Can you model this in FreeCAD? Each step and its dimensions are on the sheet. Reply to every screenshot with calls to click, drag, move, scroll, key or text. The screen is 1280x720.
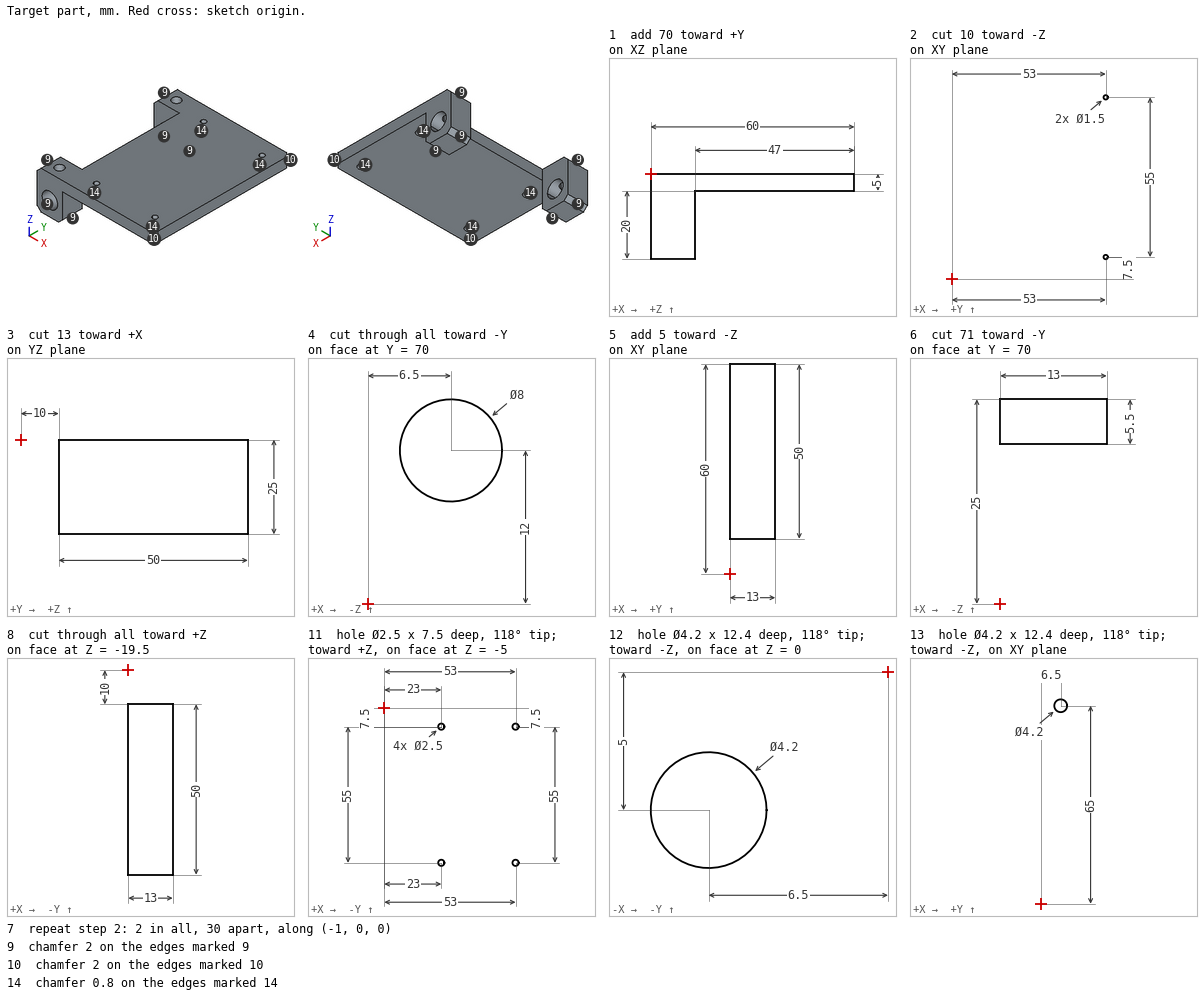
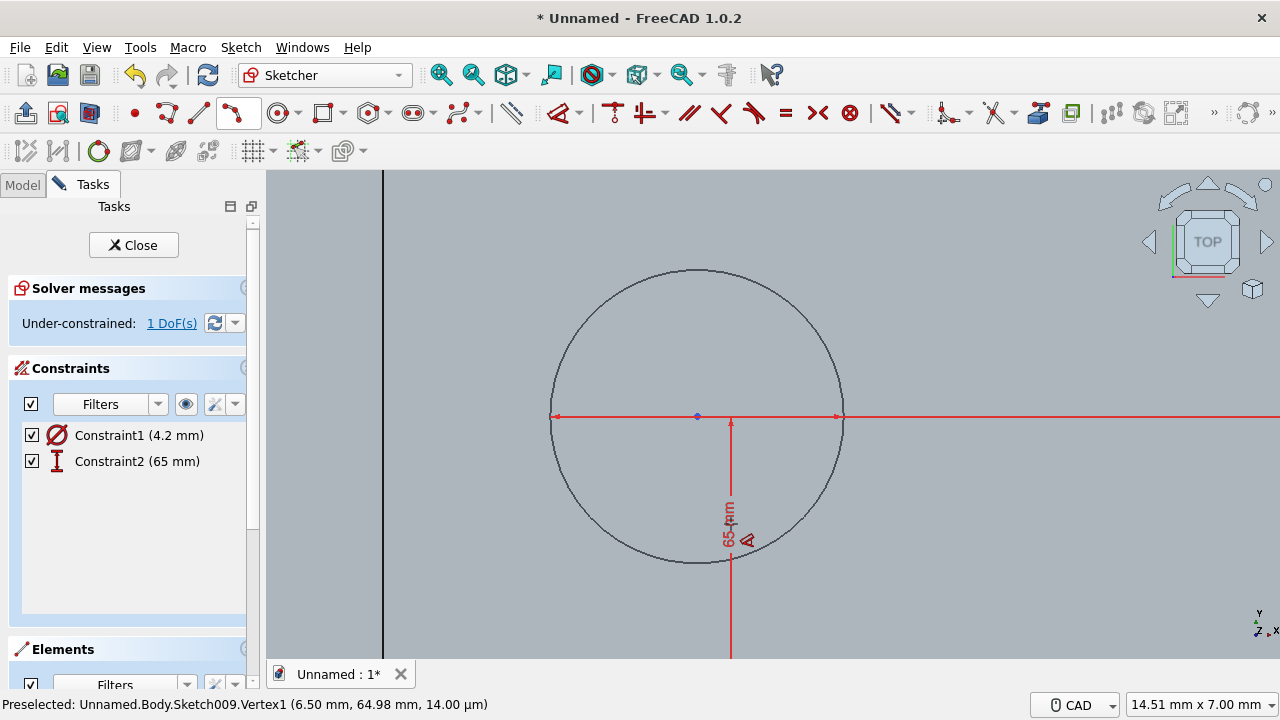
click(697, 417)
click(496, 383)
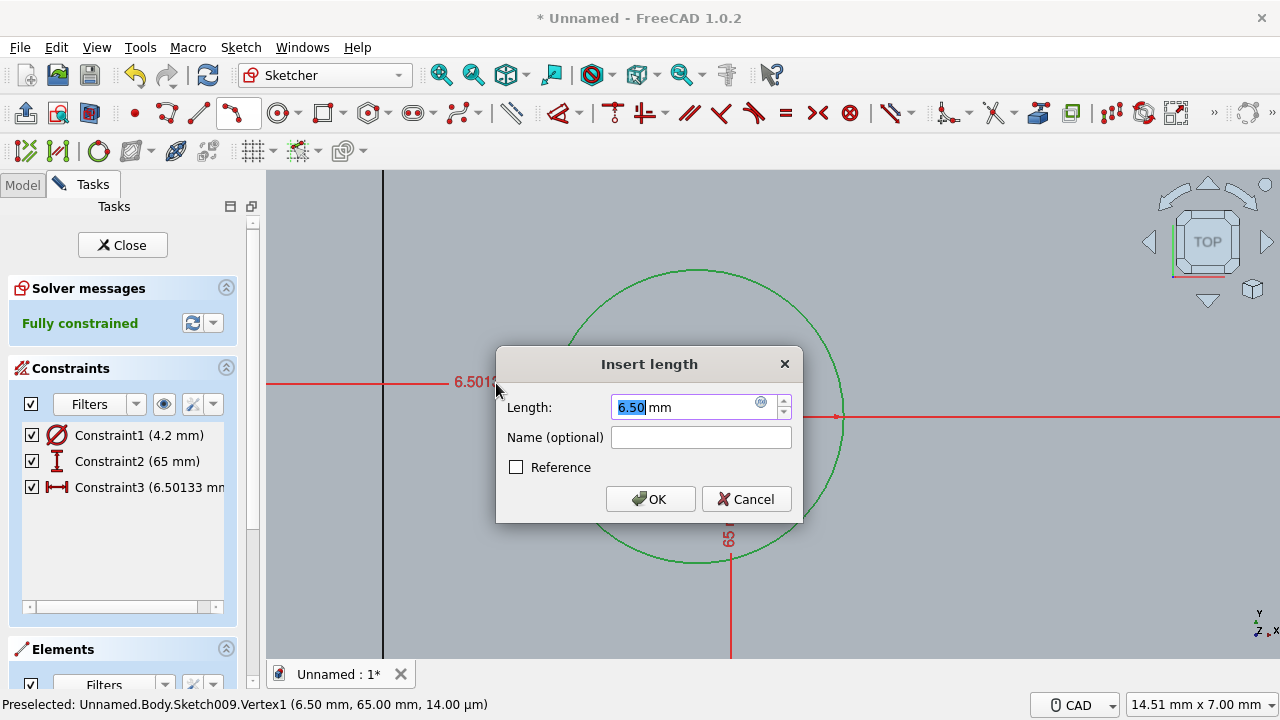
text(6.5)
key(Return)
key(Escape)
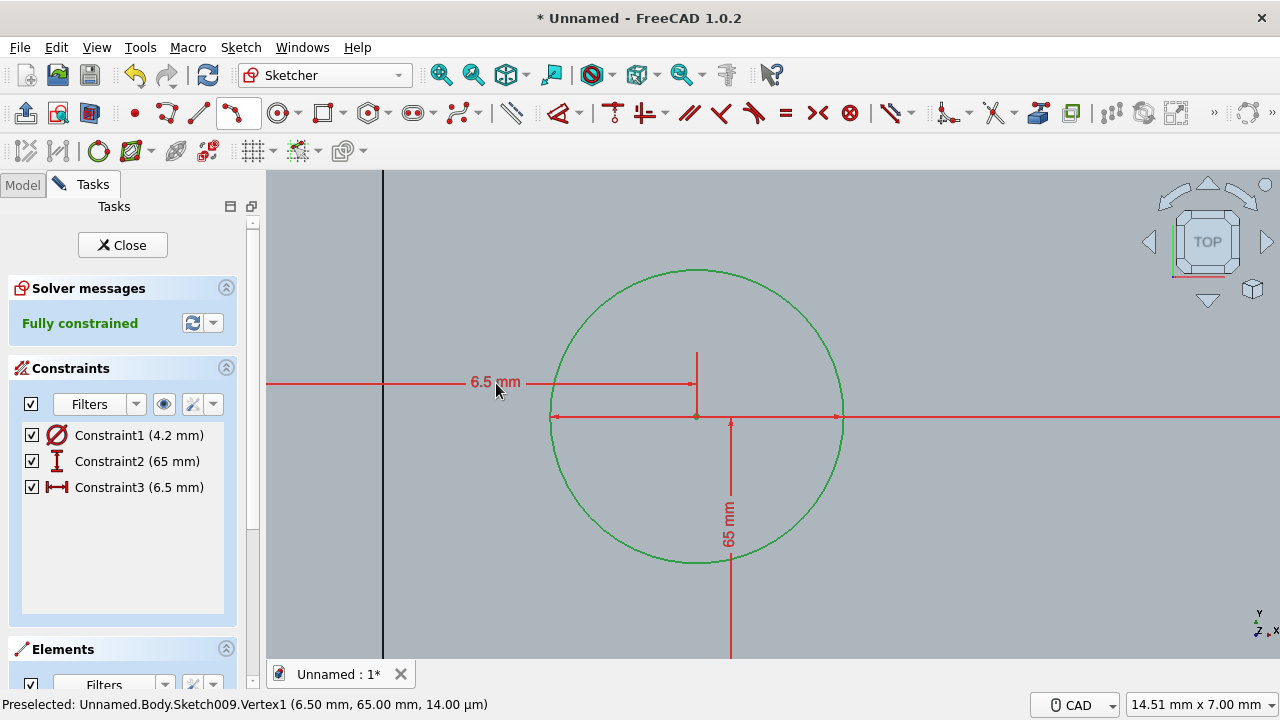
click(123, 245)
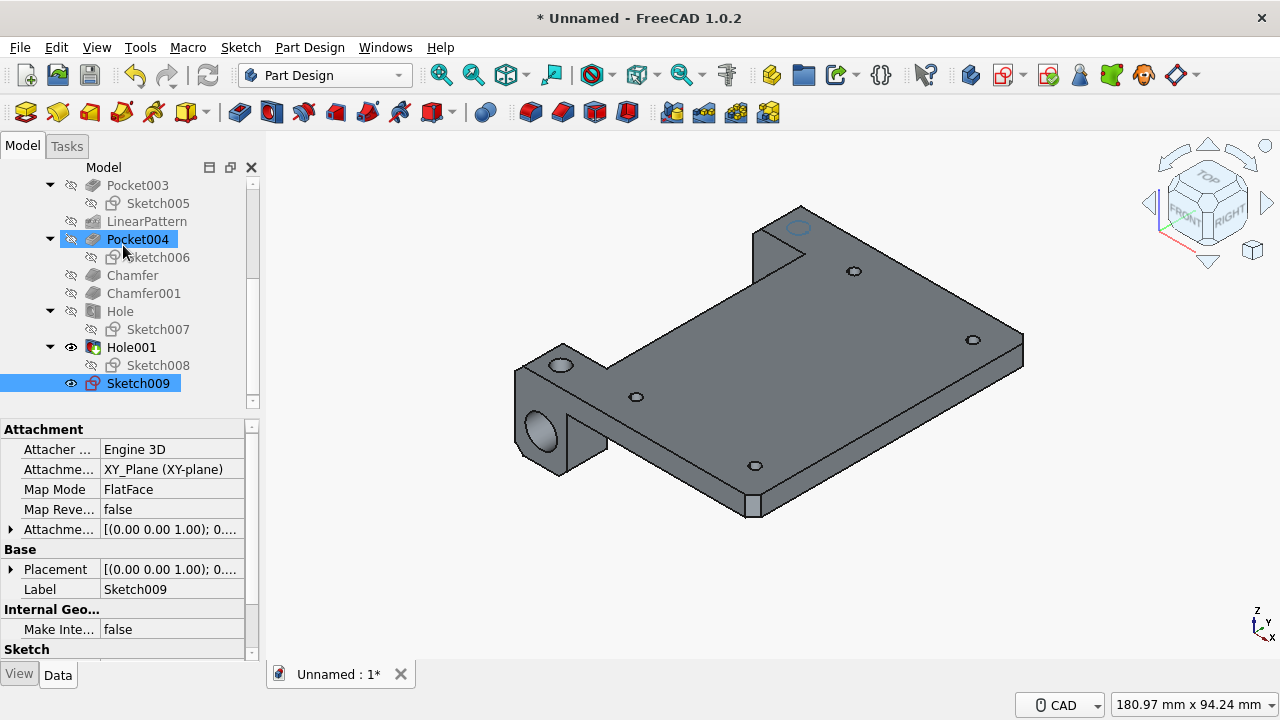
click(272, 112)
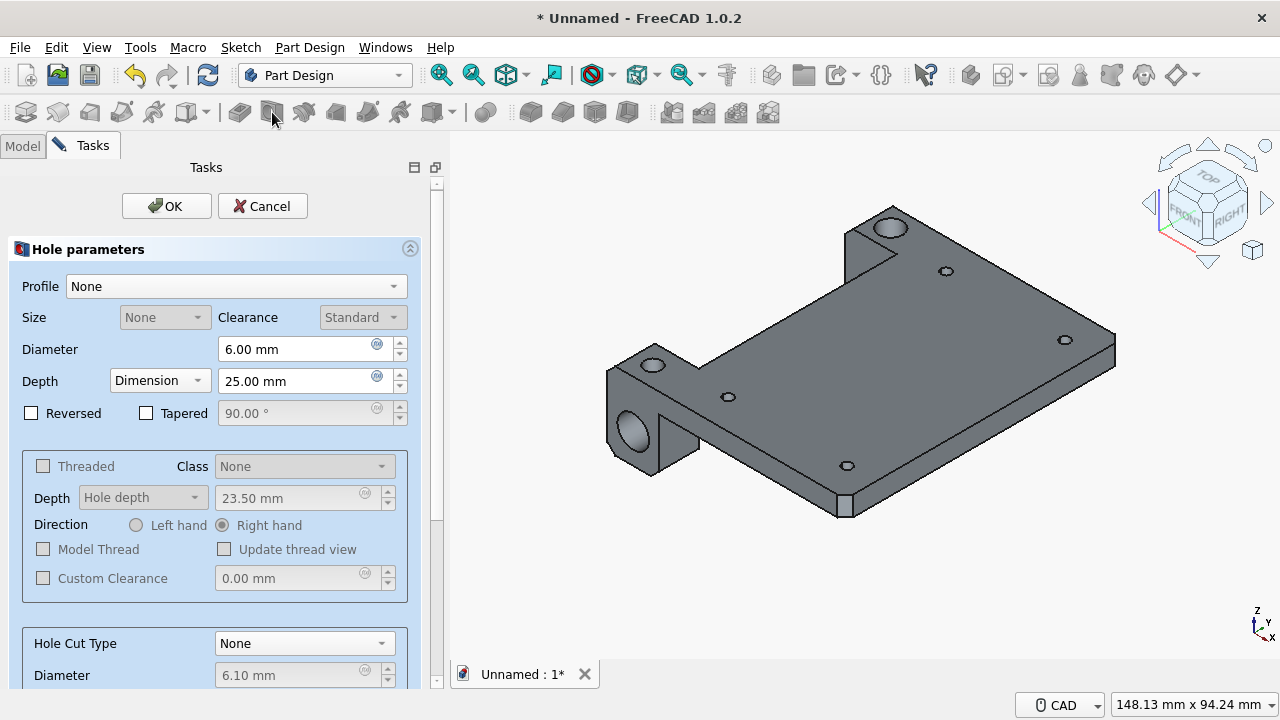
triple_click(305, 349)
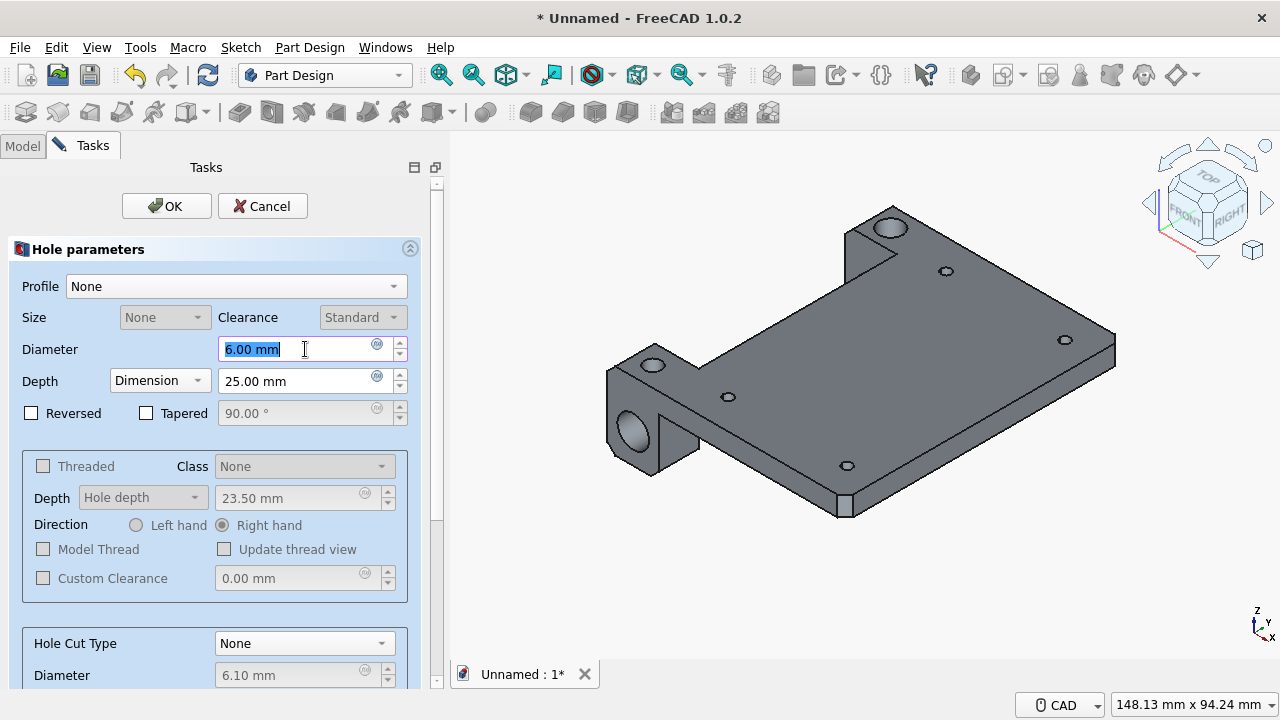
text(4.2)
key(Tab)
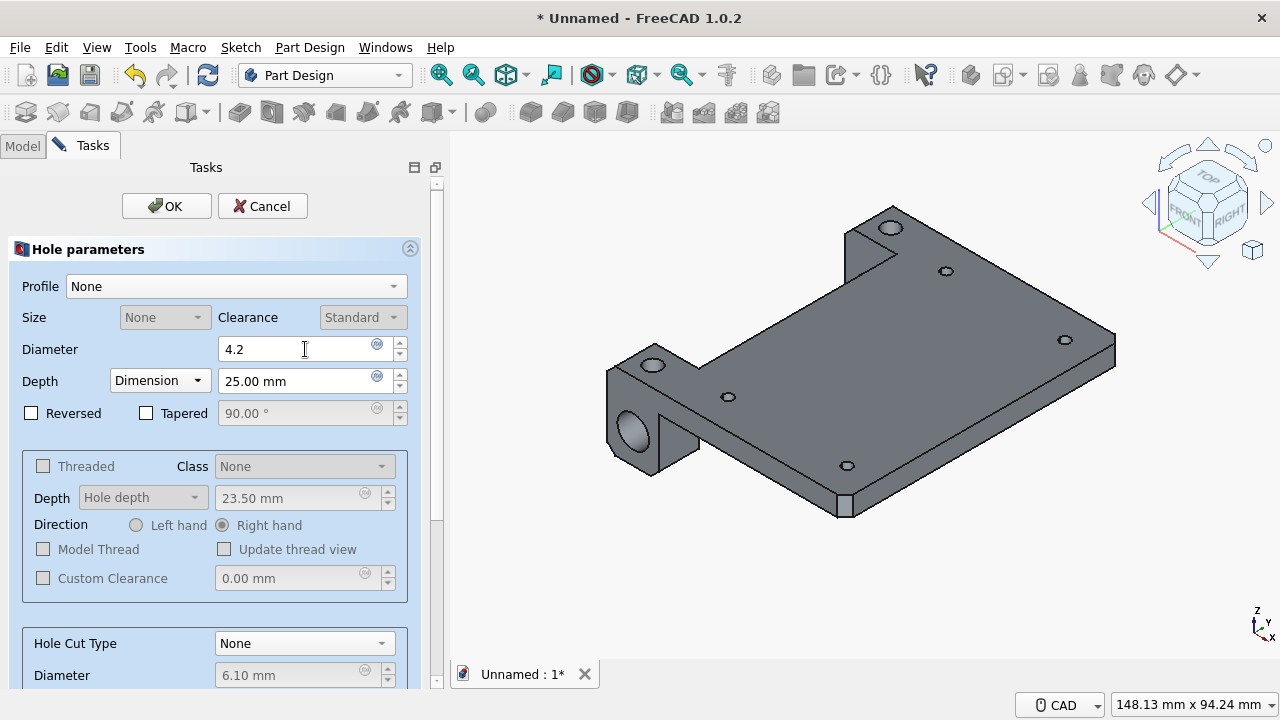
triple_click(305, 381)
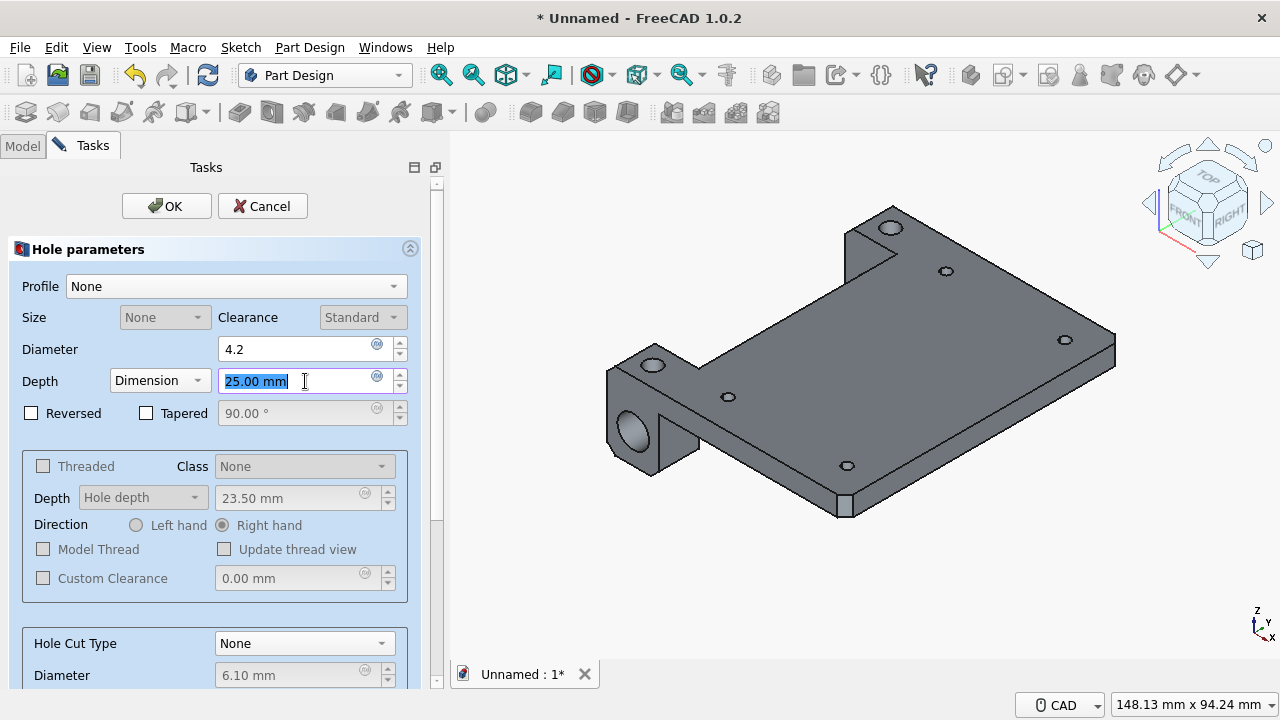
text(12.4)
key(Tab)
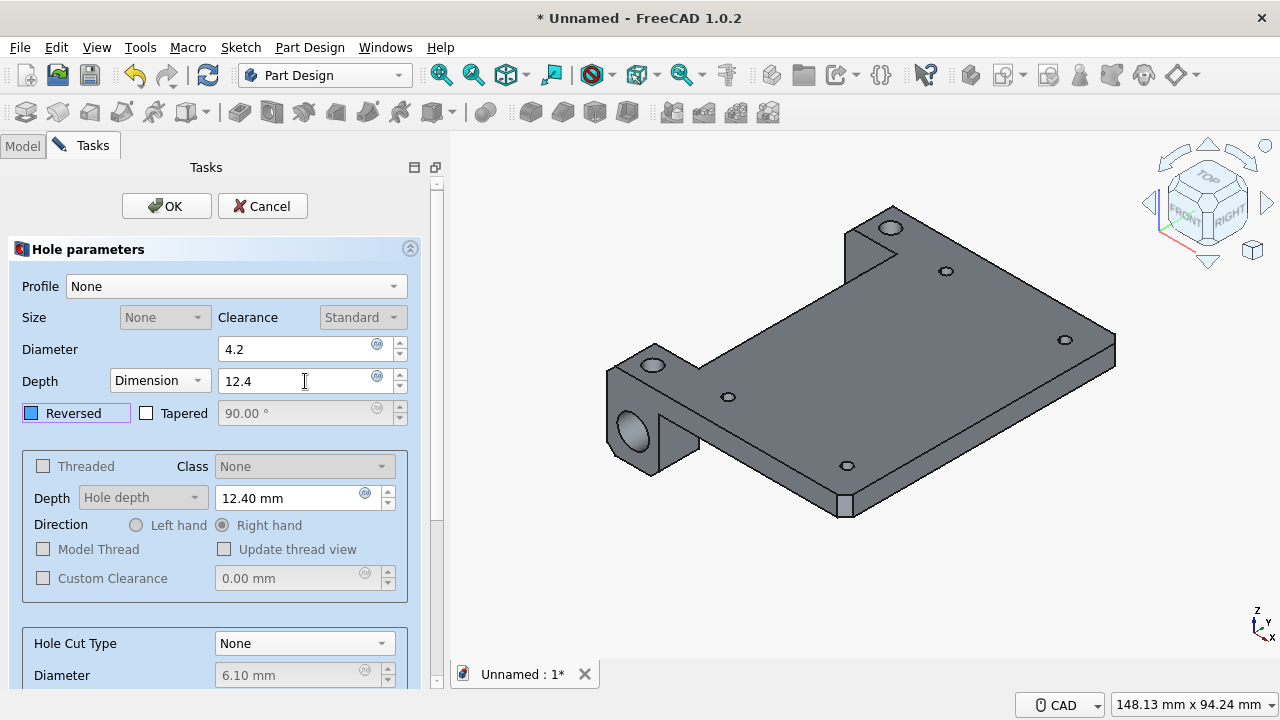
click(167, 206)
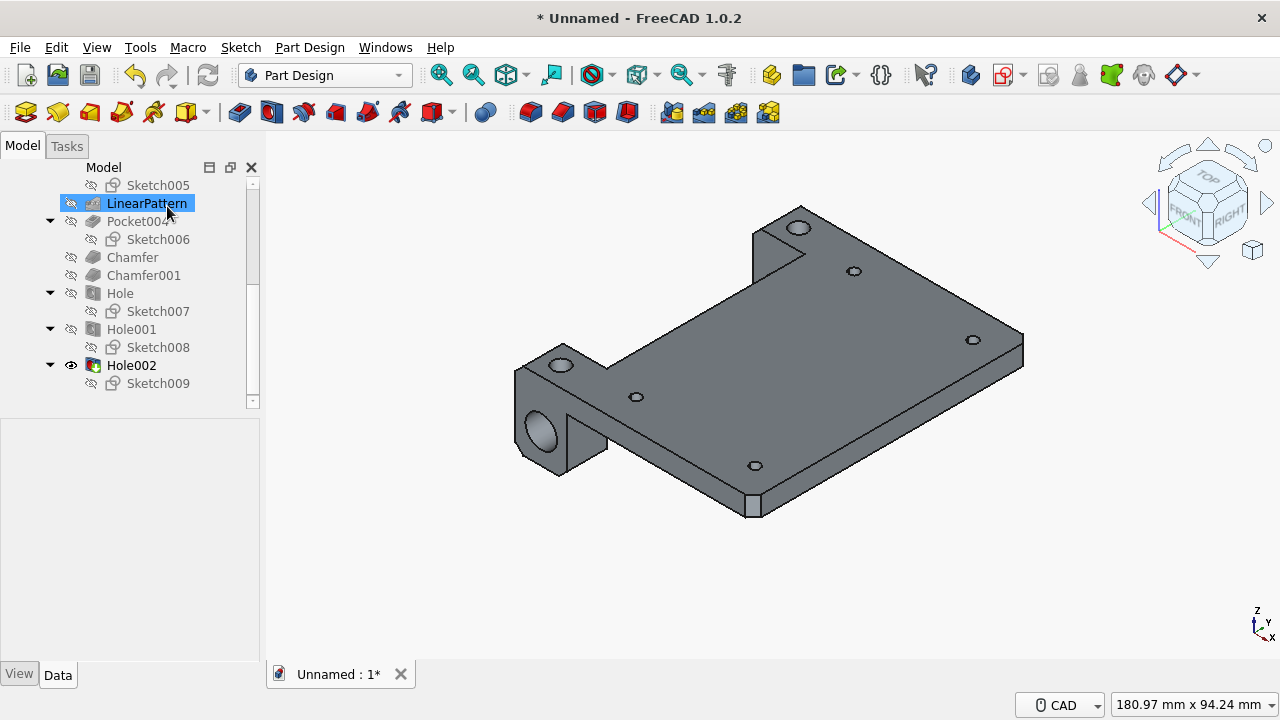
key(2)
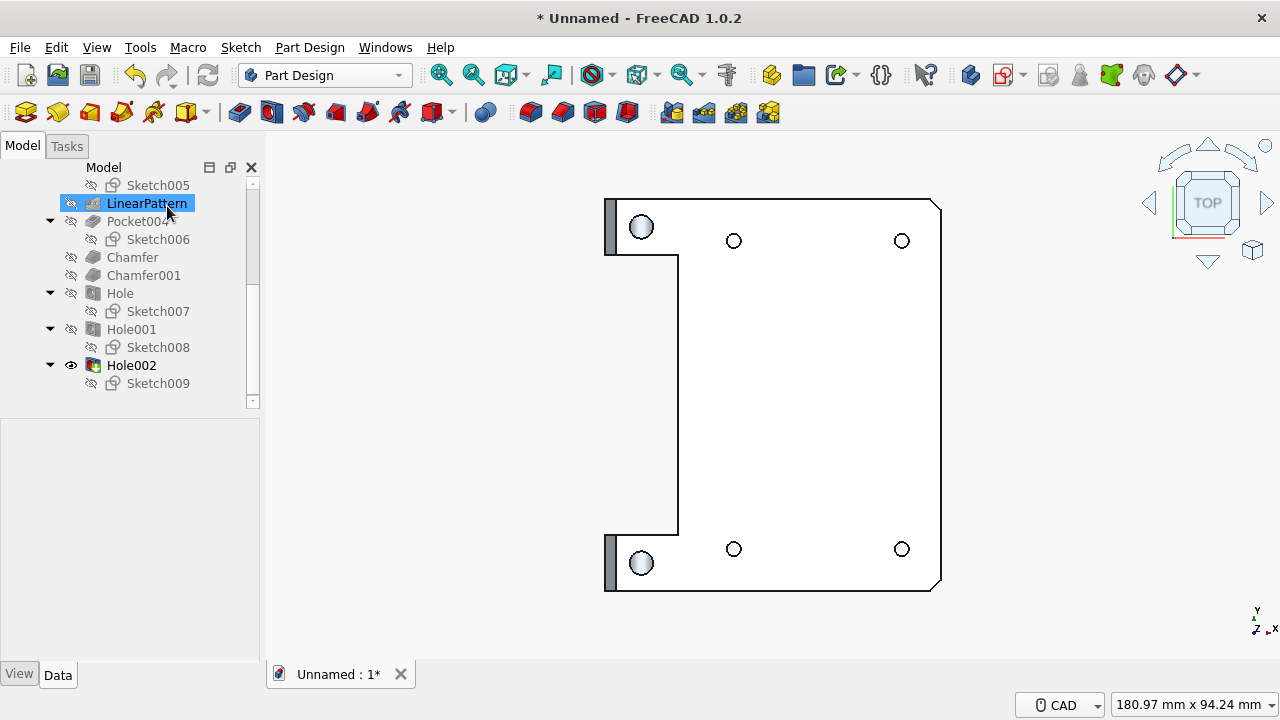
key(0)